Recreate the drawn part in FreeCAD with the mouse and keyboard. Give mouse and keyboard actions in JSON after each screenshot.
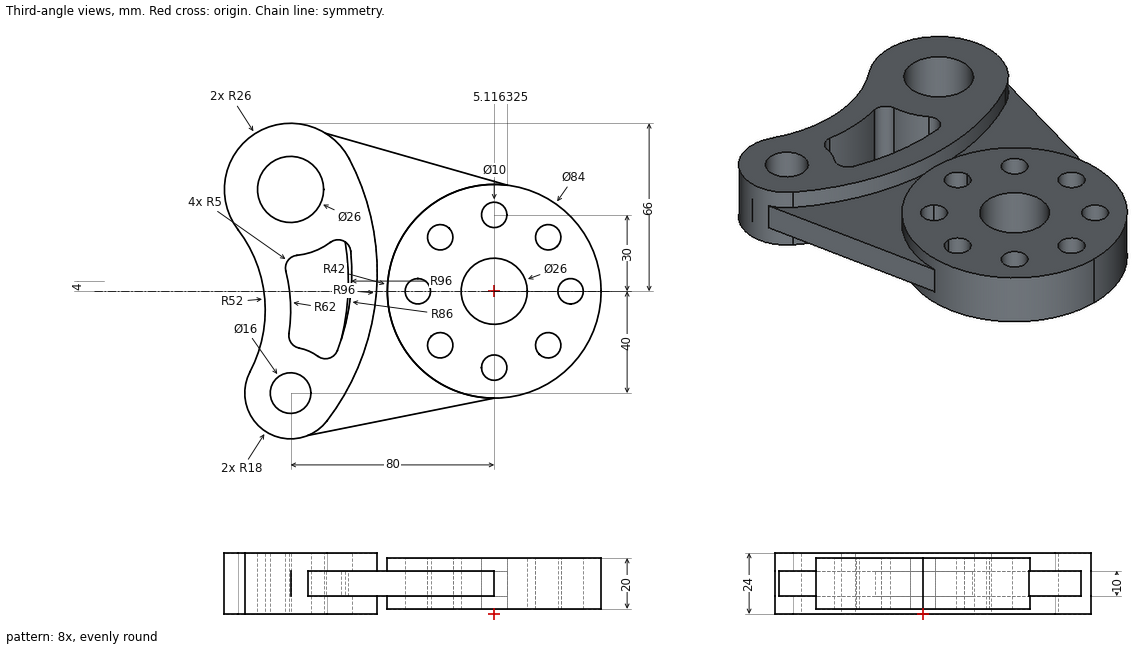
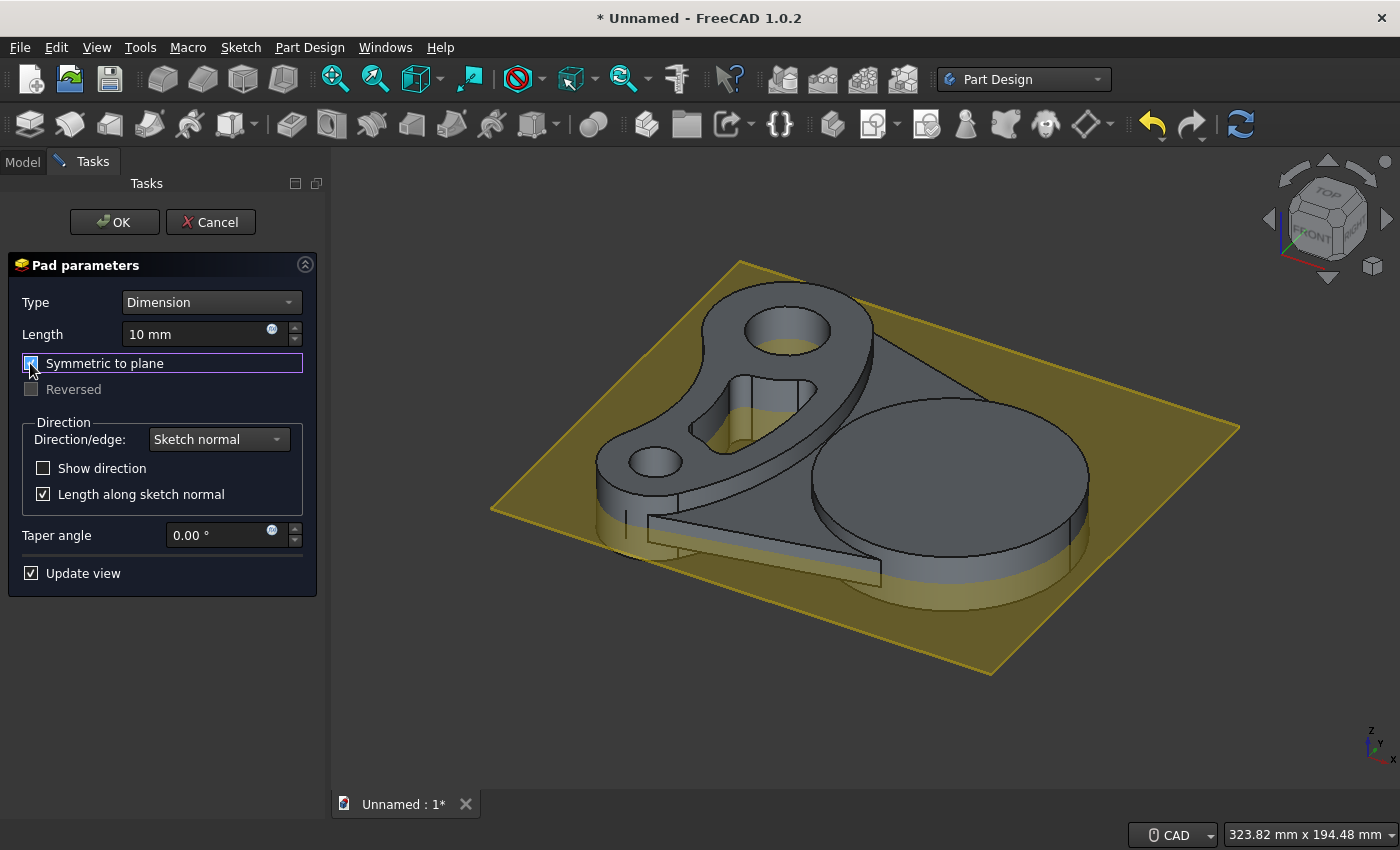
{"action": "left_click", "coordinate": [115, 222]}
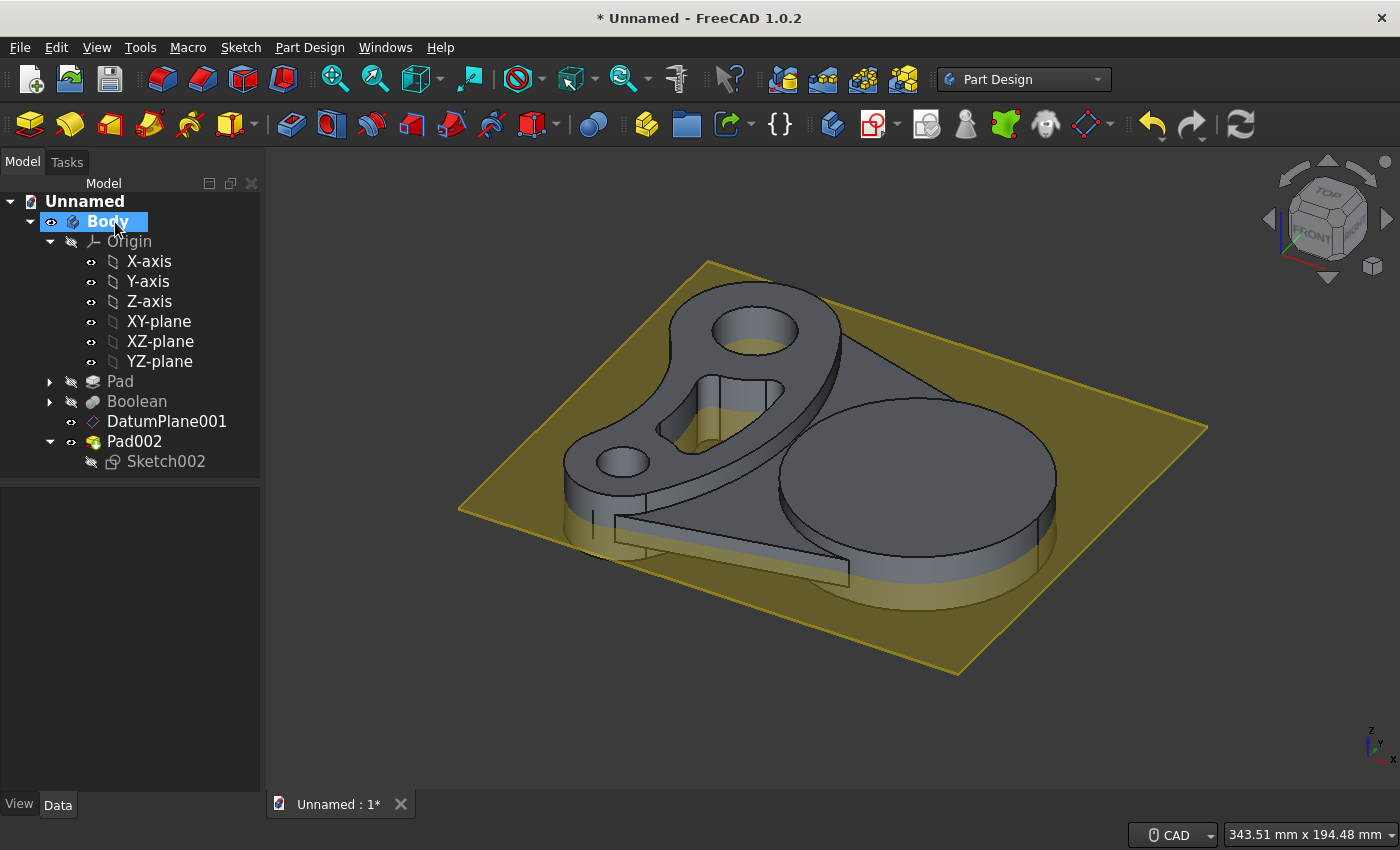
{"action": "left_click", "coordinate": [116, 422]}
{"action": "key", "text": "space"}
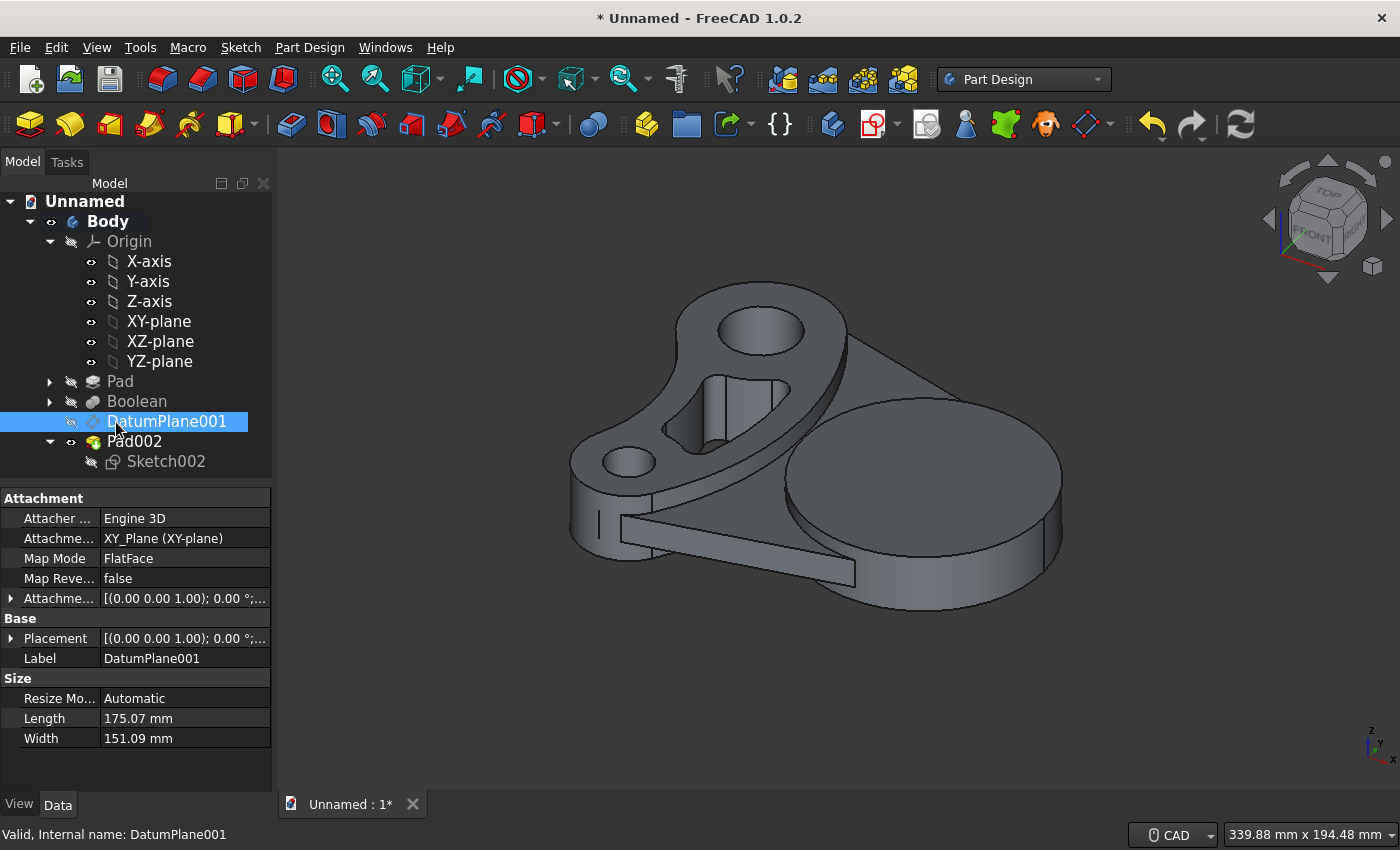
{"action": "left_click", "coordinate": [924, 477]}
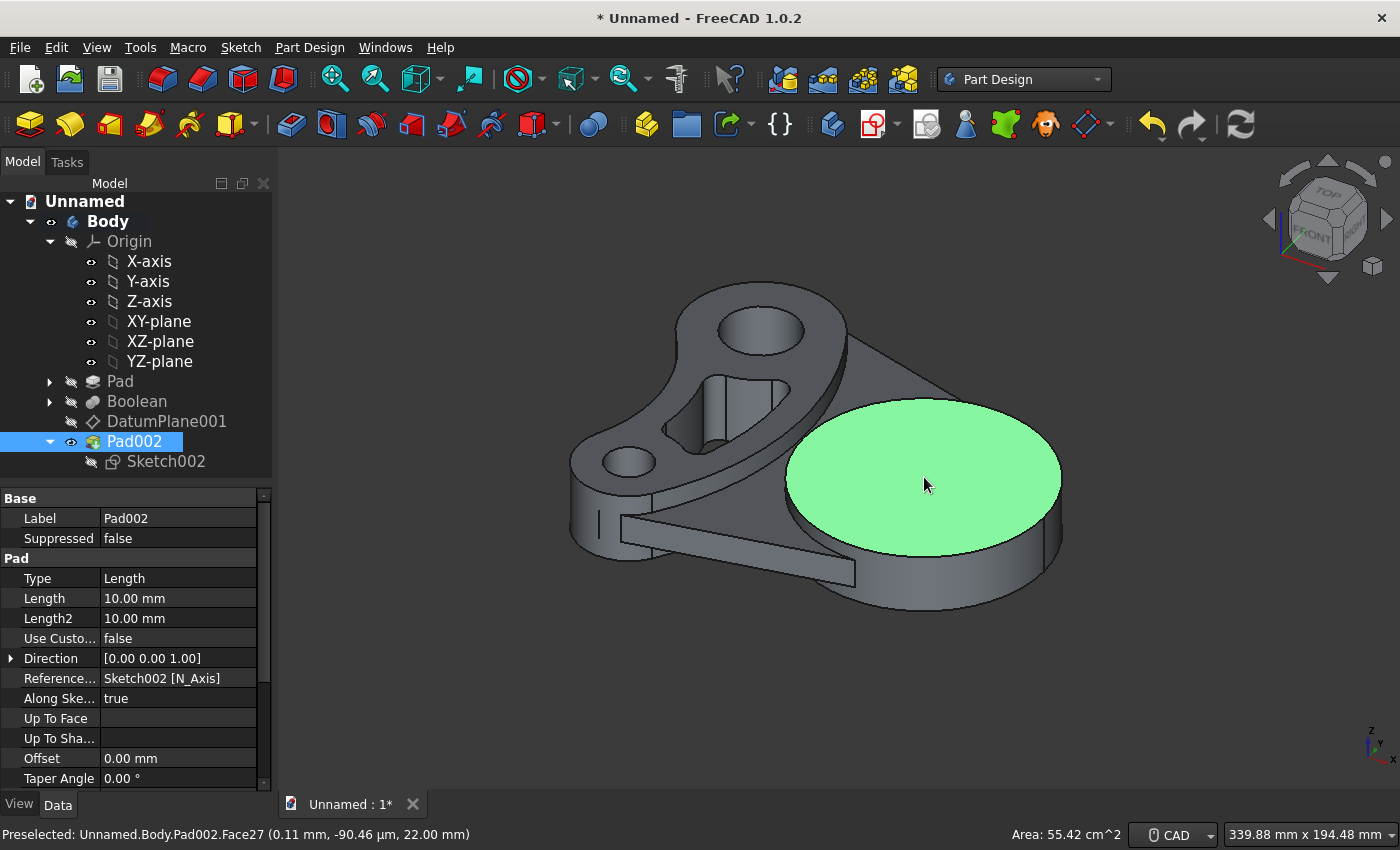
{"action": "left_click", "coordinate": [874, 124]}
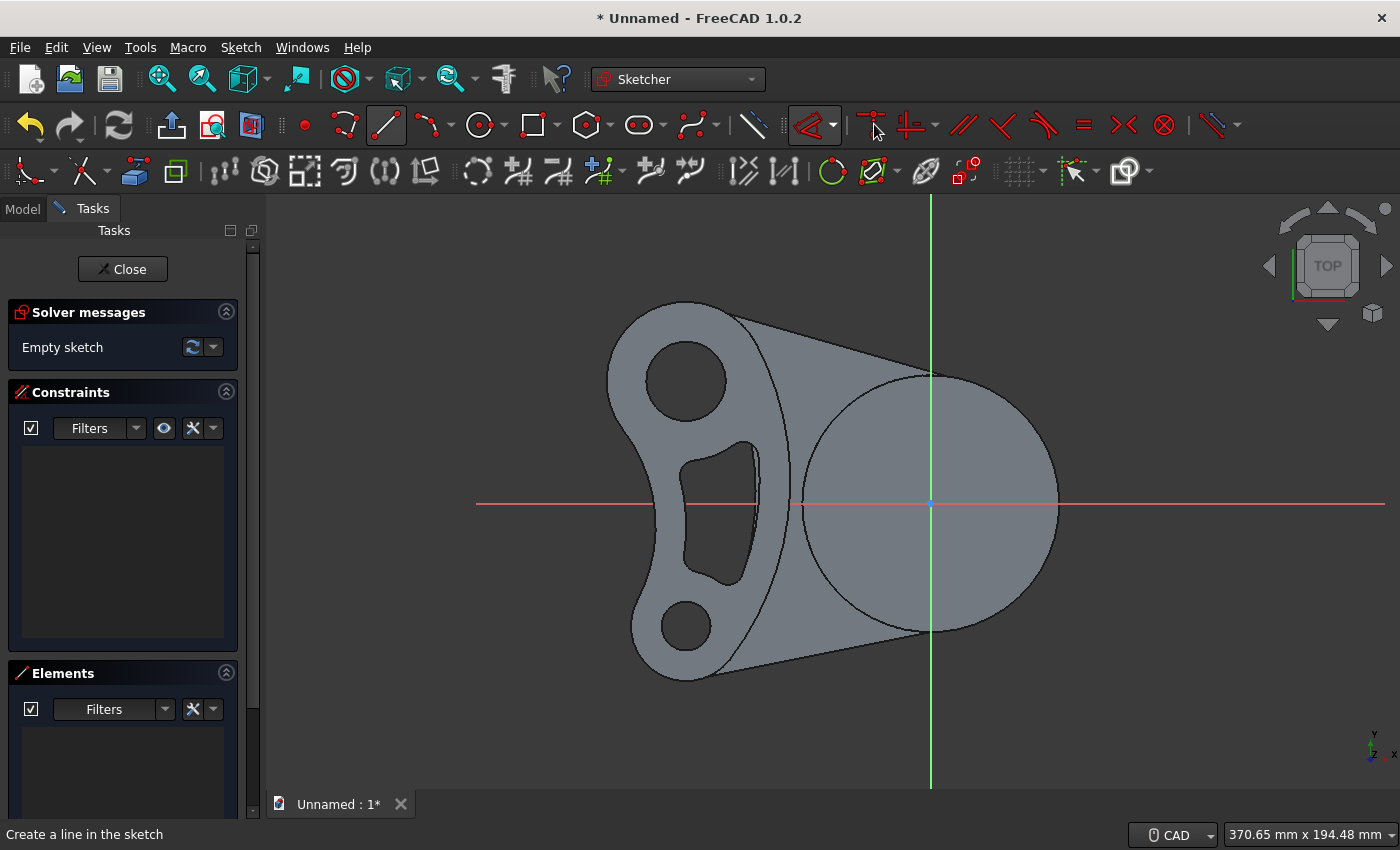
{"action": "scroll", "coordinate": [973, 507], "scroll_direction": "up", "scroll_amount": 8}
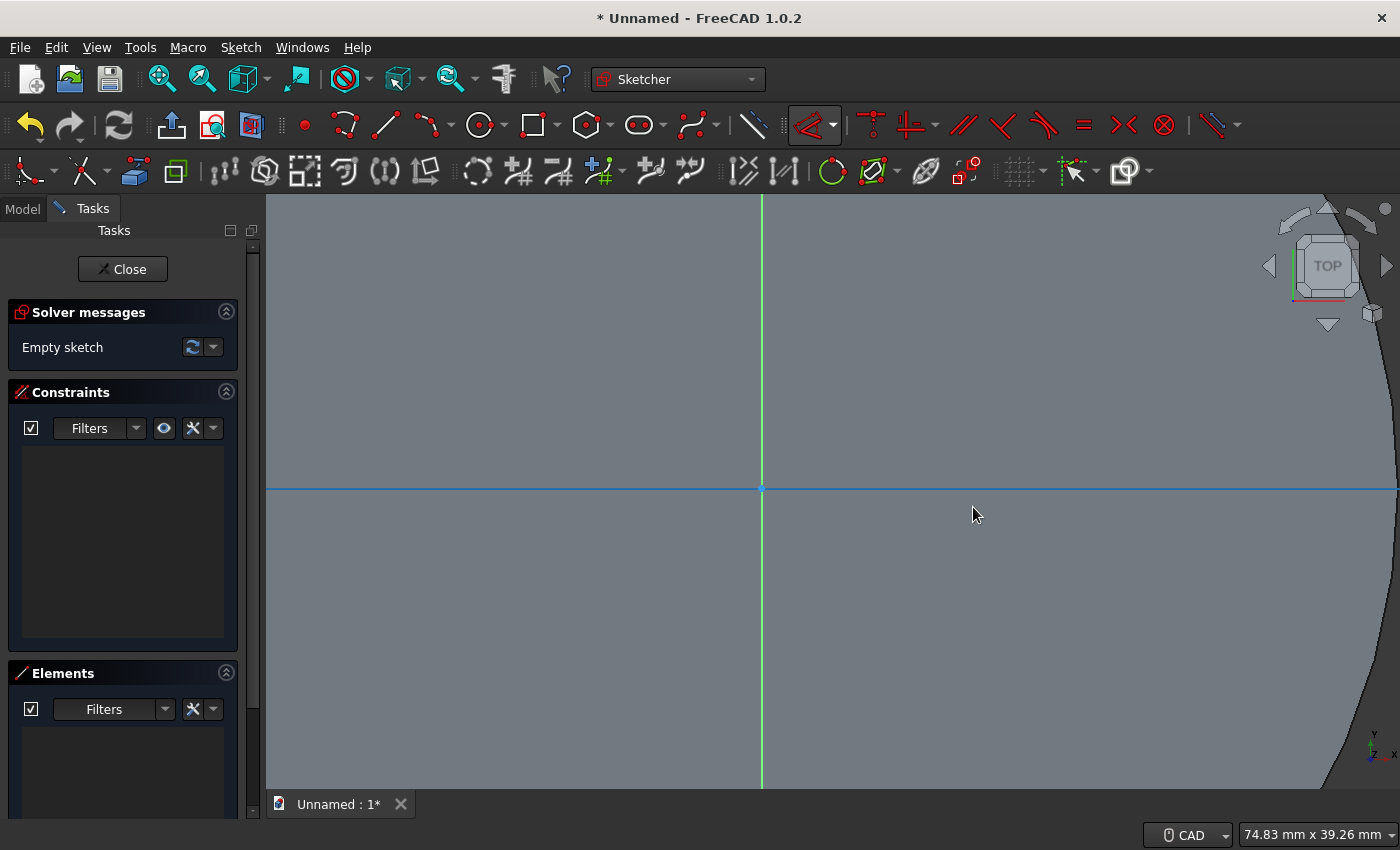
{"action": "left_click", "coordinate": [480, 126]}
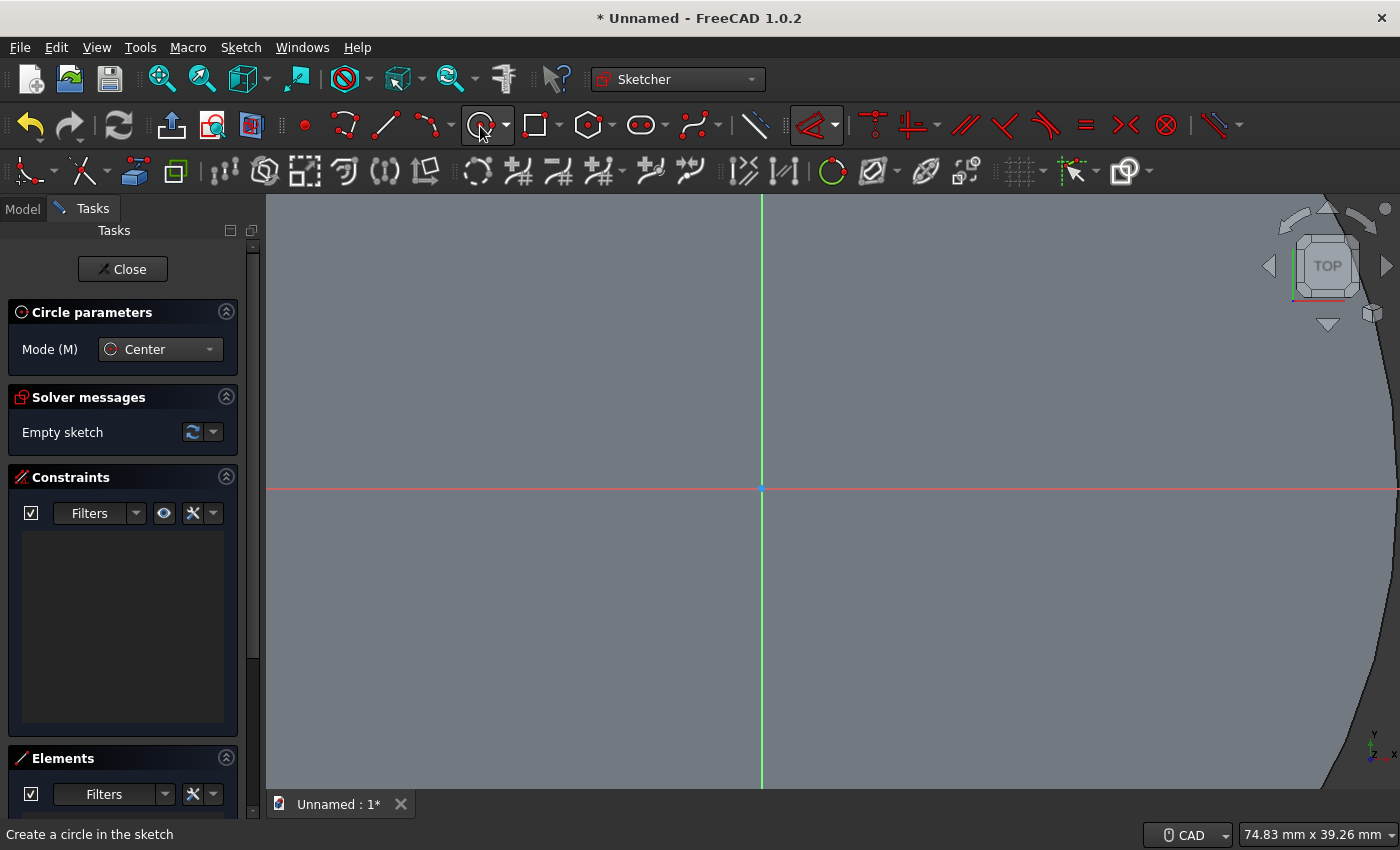
{"action": "left_click", "coordinate": [762, 489]}
{"action": "left_click", "coordinate": [901, 349]}
{"action": "key", "text": "Escape"}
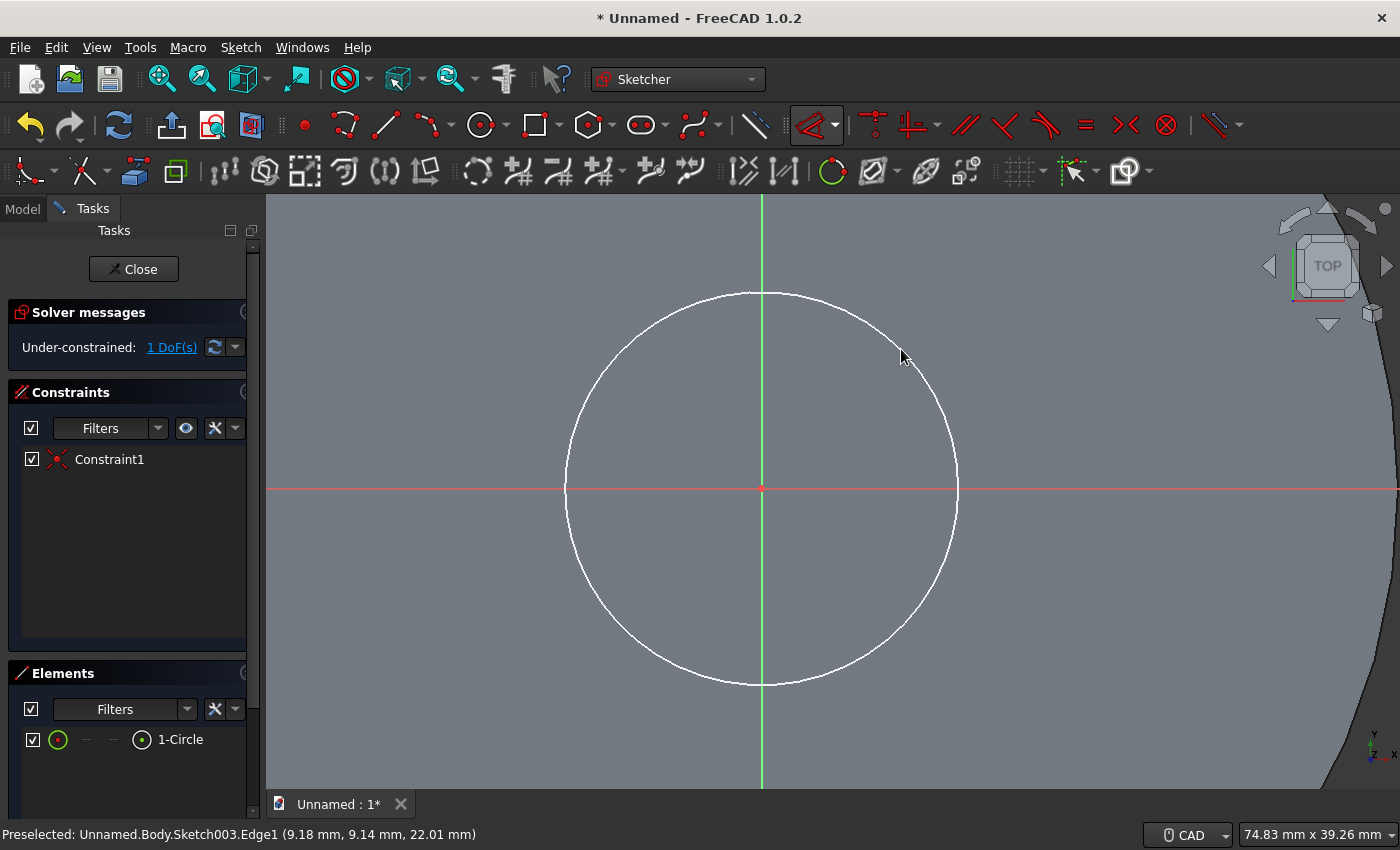
{"action": "left_click", "coordinate": [900, 349]}